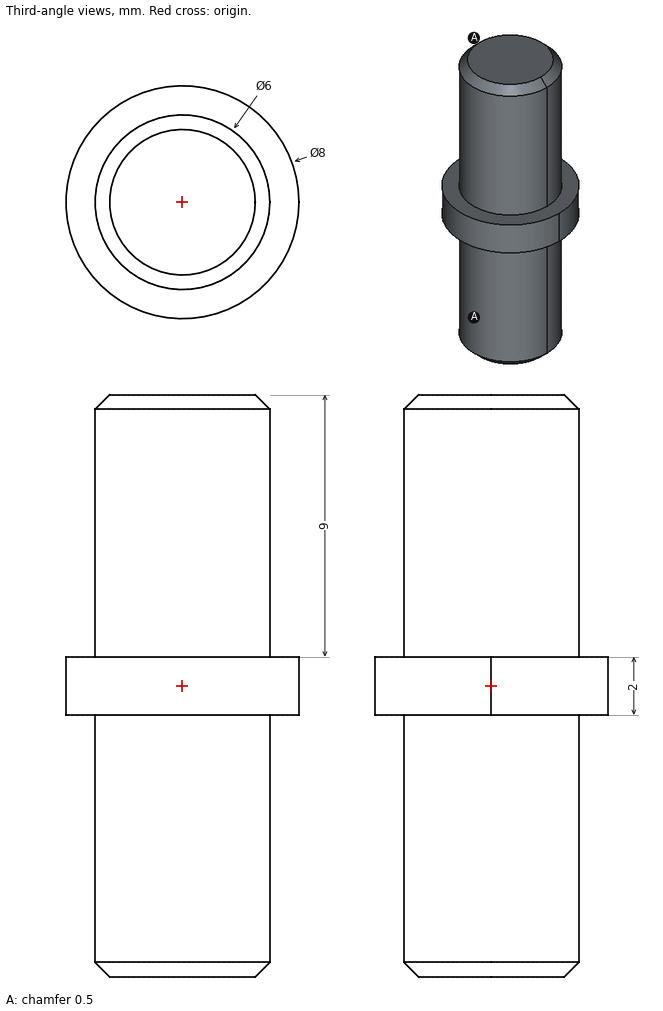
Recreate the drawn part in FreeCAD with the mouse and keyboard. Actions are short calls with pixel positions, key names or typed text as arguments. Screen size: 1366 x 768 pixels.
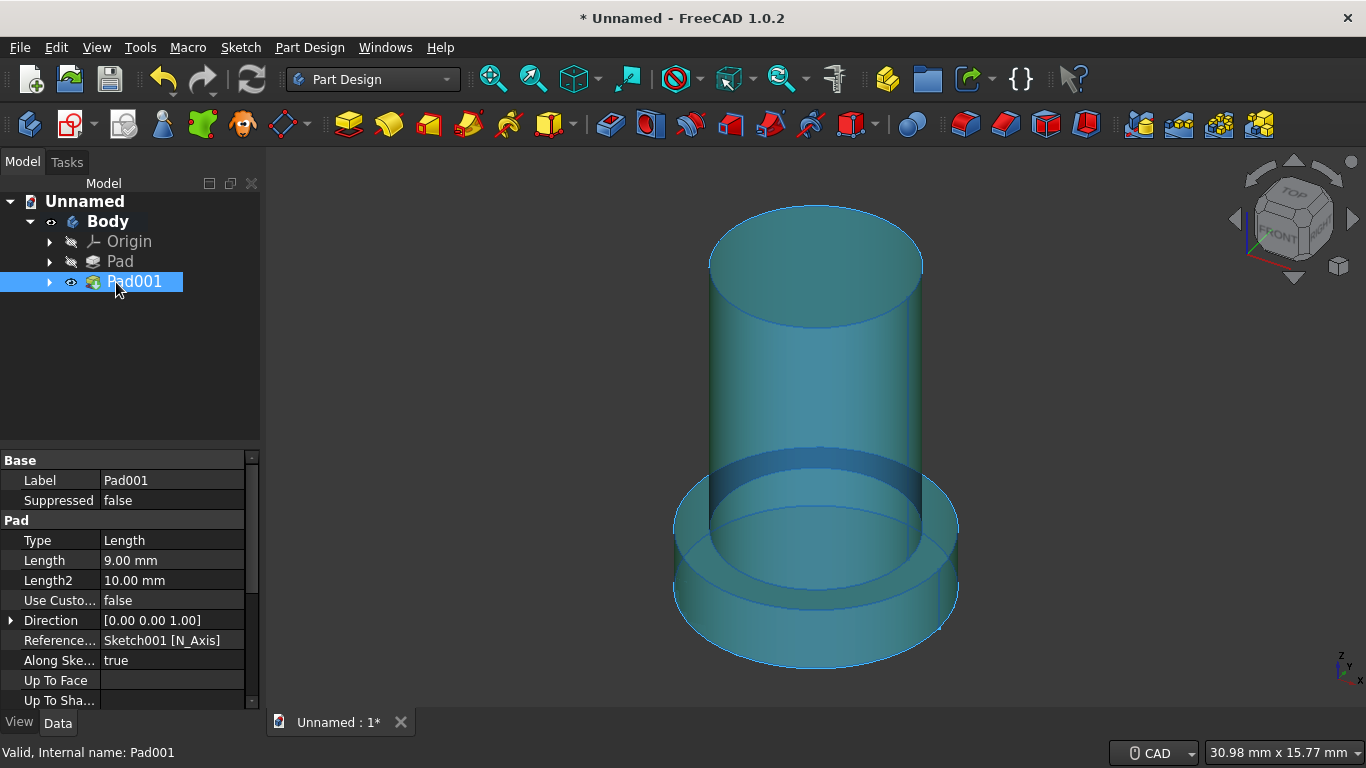
click(1140, 124)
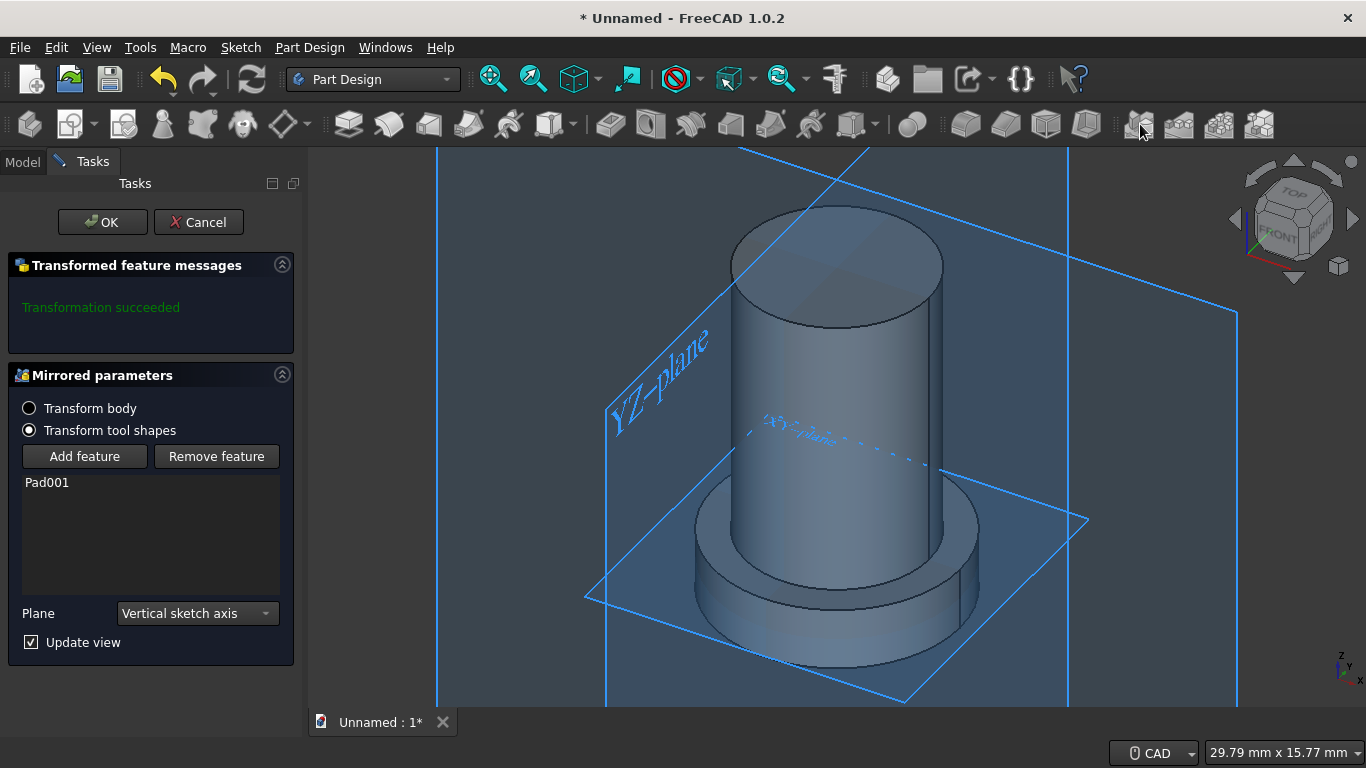
click(198, 614)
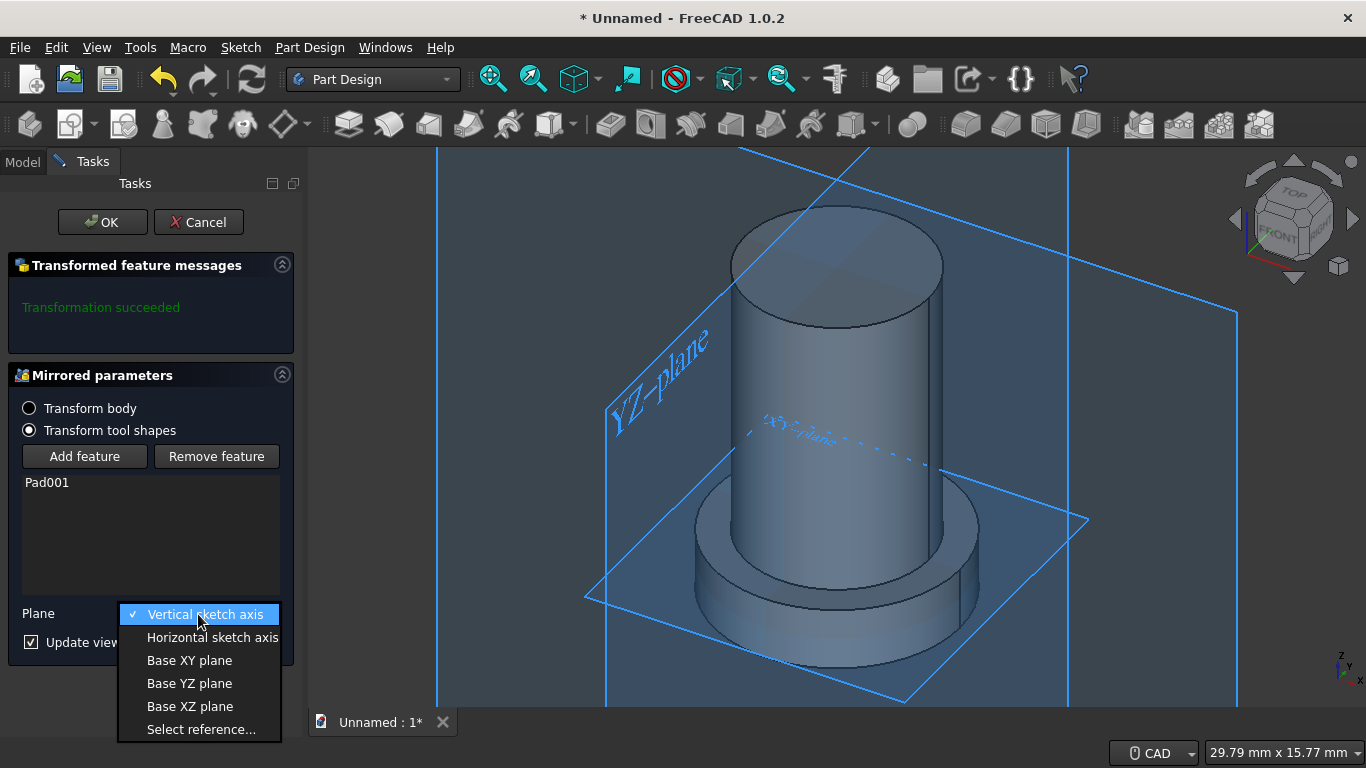
click(198, 660)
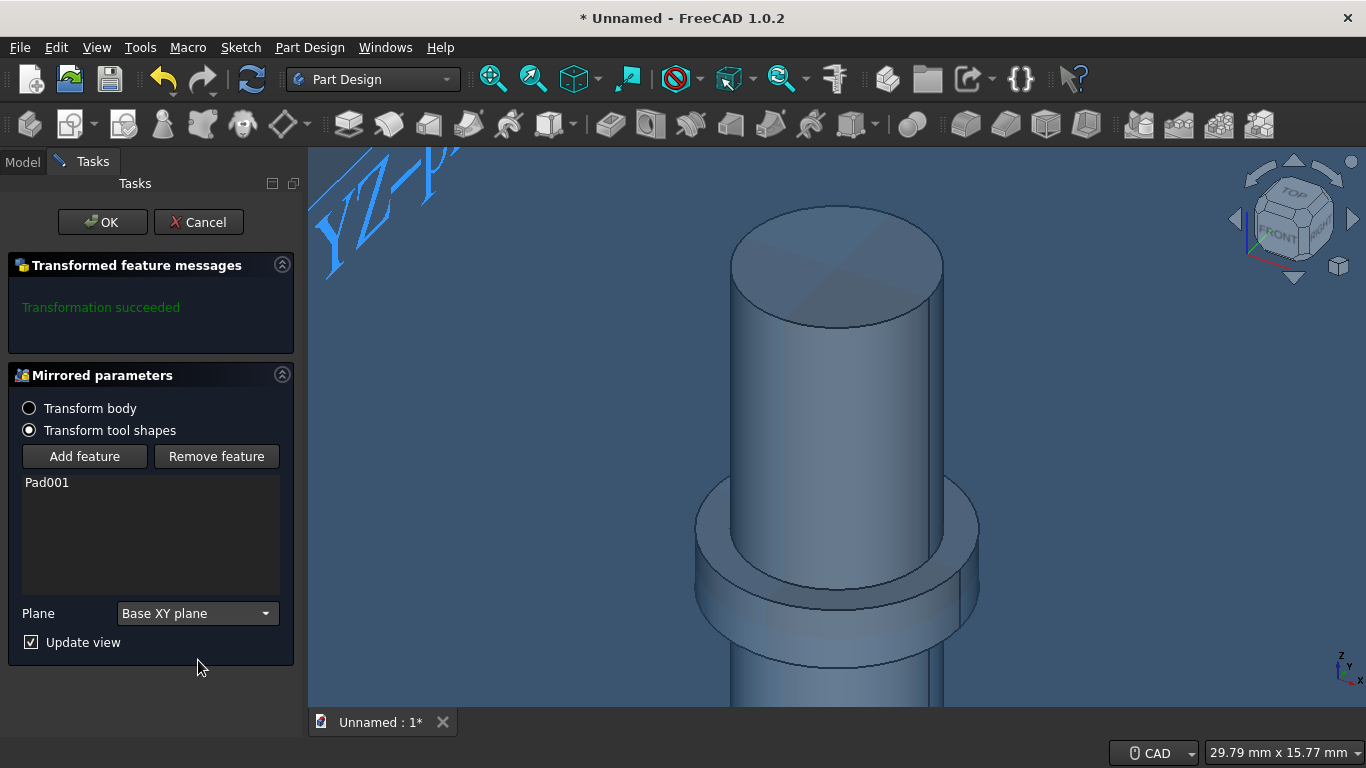
click(103, 222)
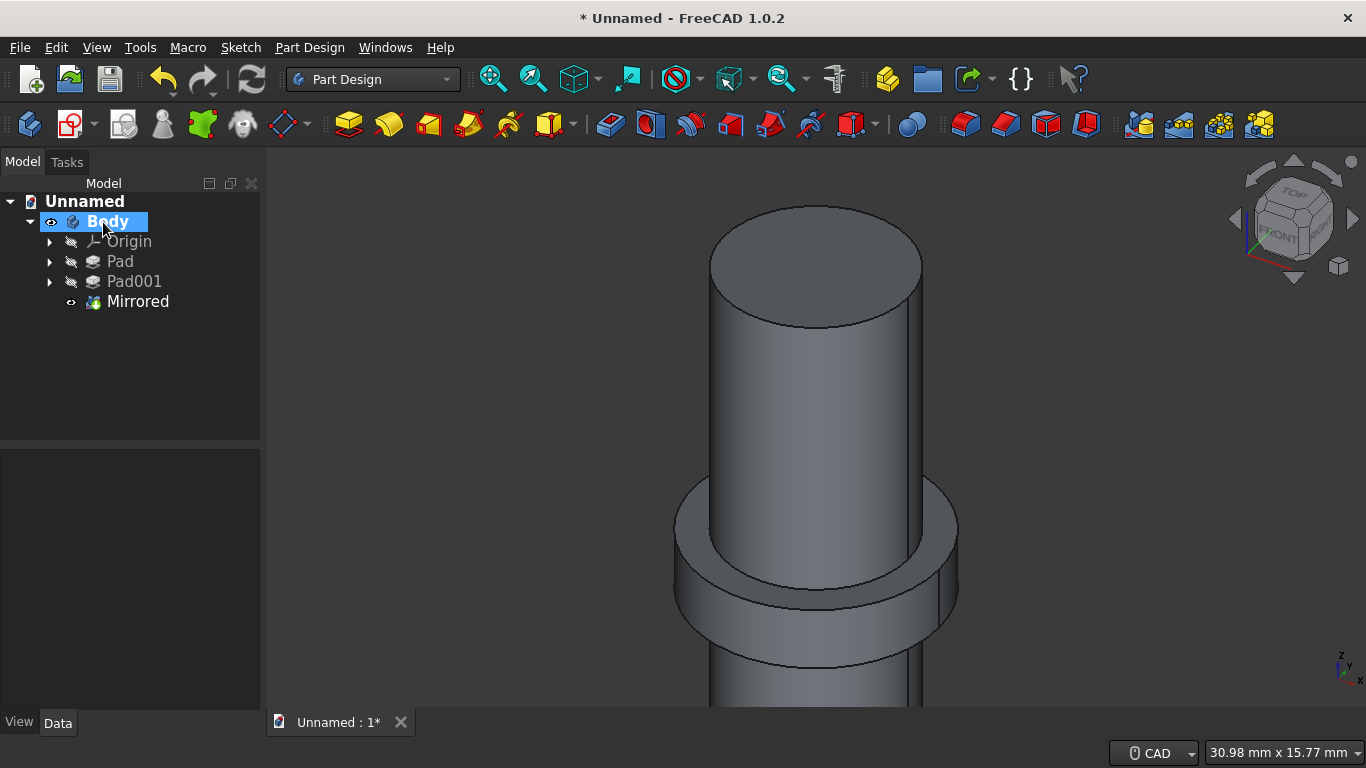
click(494, 80)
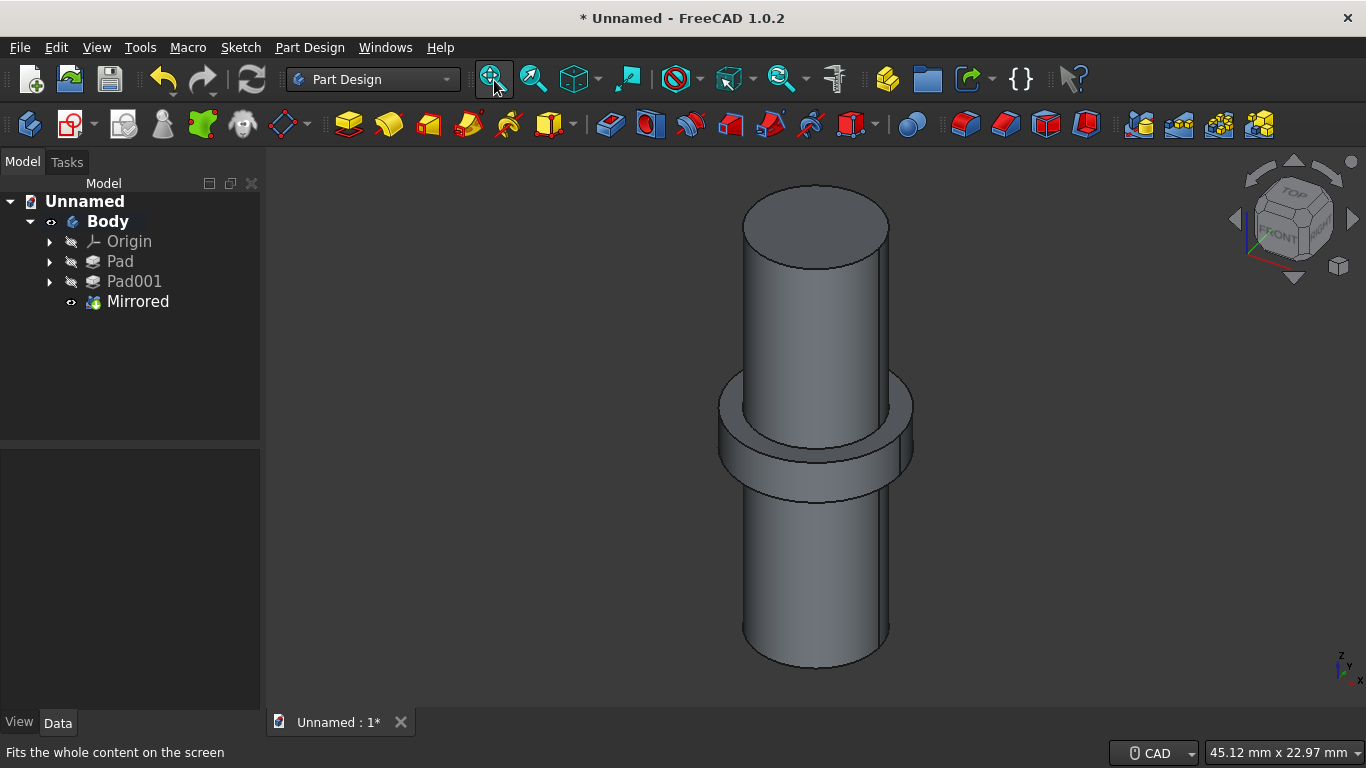
click(743, 231)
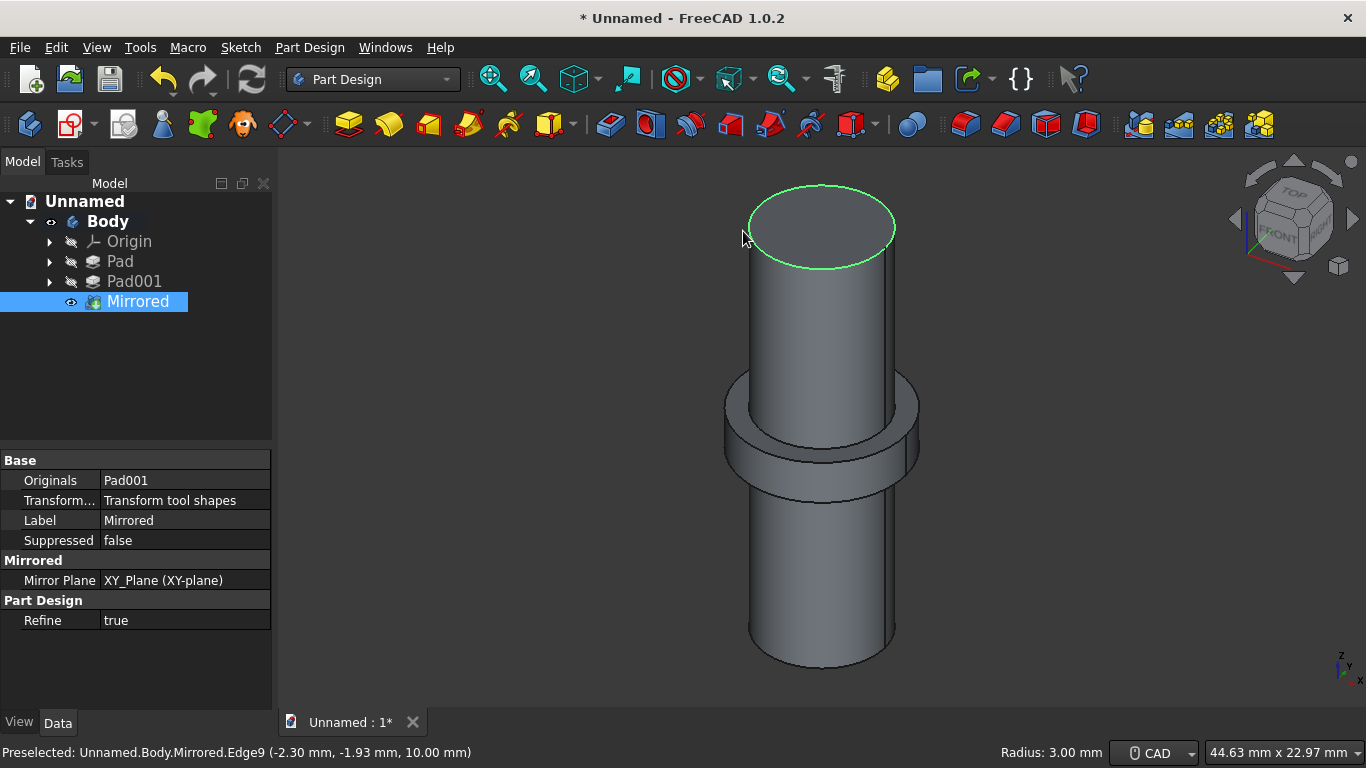
key(0)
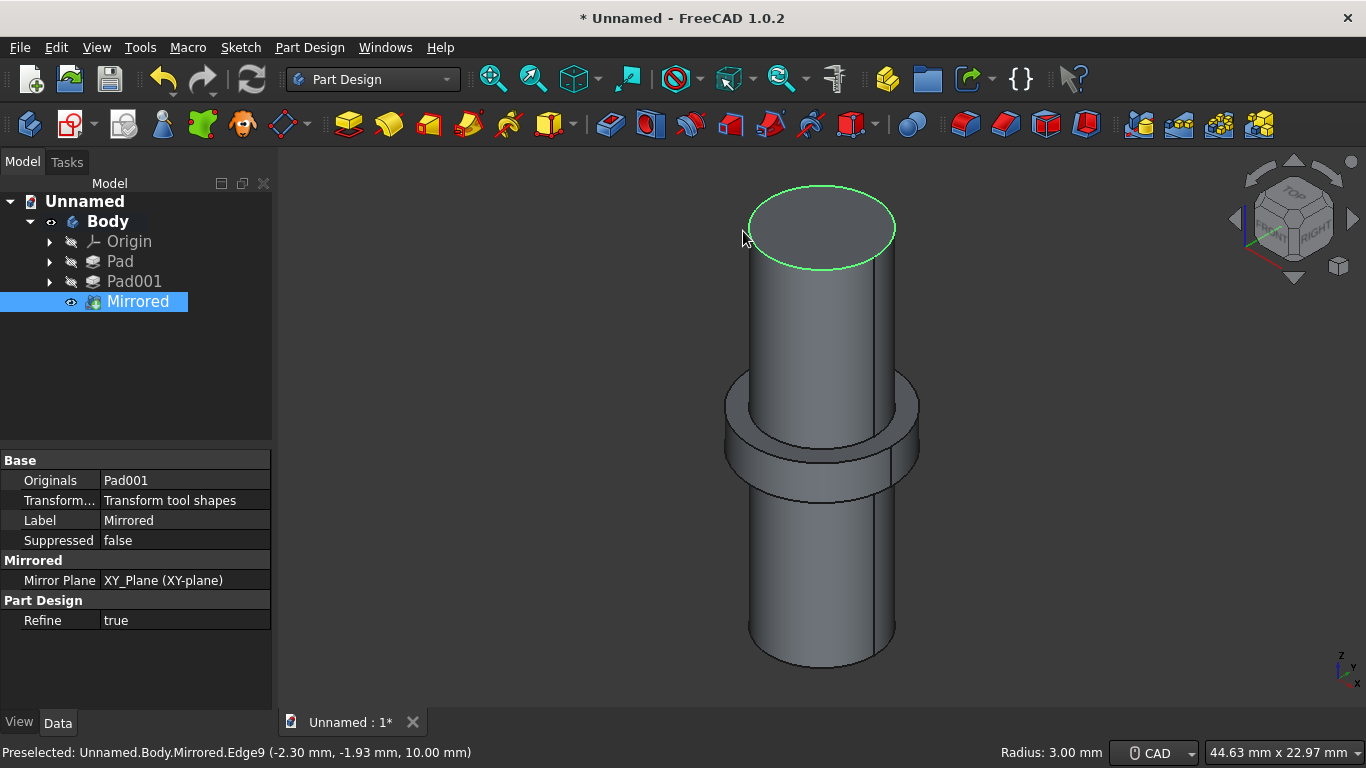
key(2)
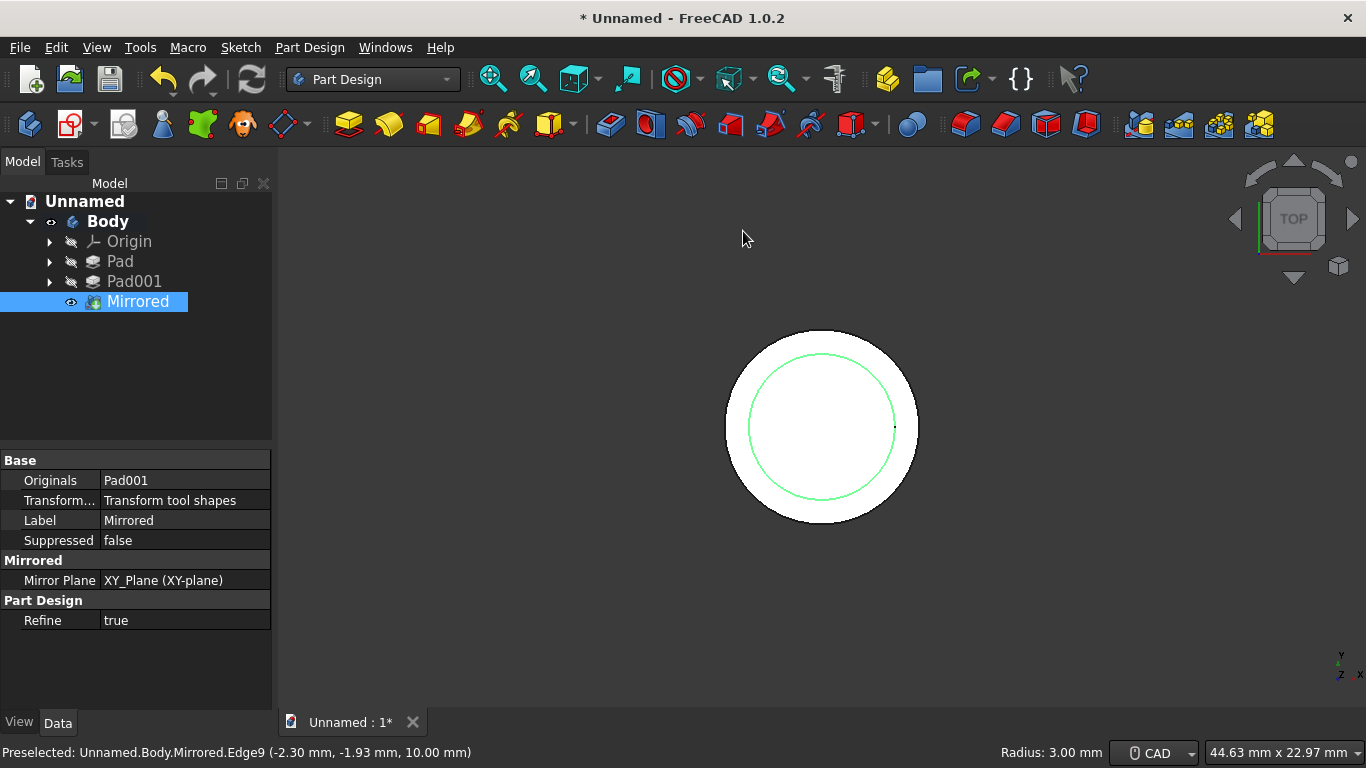
key(v)
key(f)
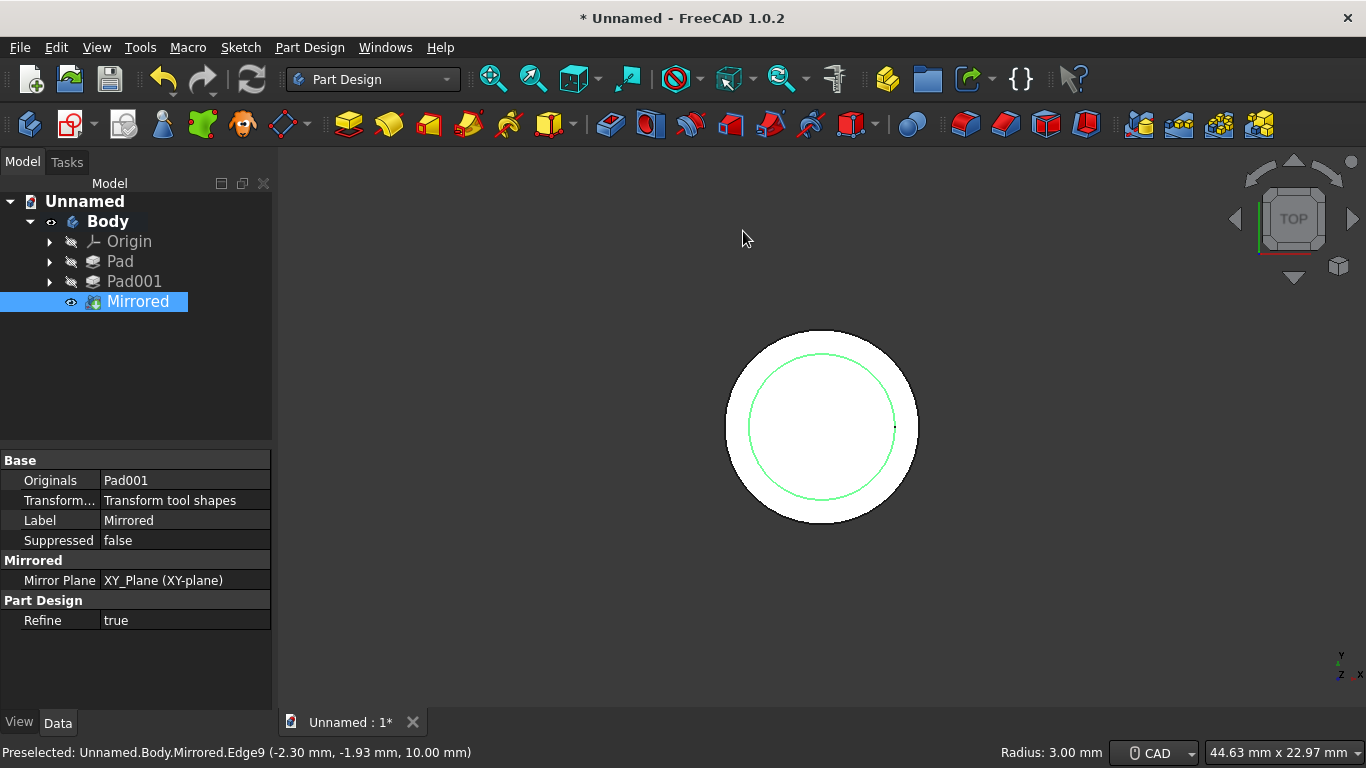
key(1)